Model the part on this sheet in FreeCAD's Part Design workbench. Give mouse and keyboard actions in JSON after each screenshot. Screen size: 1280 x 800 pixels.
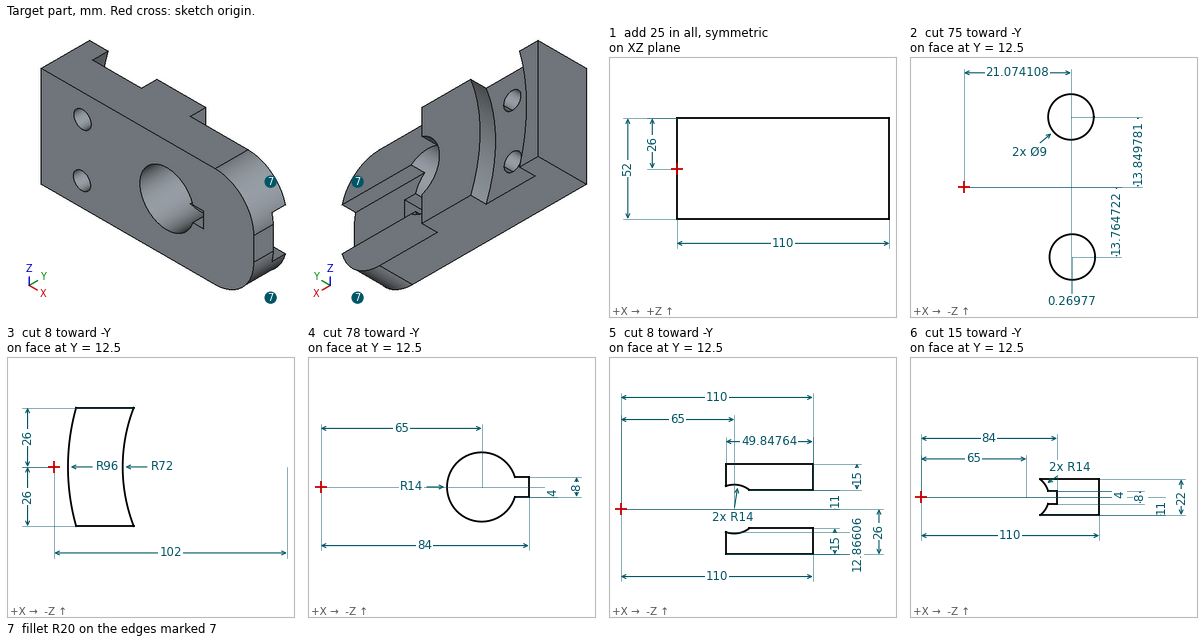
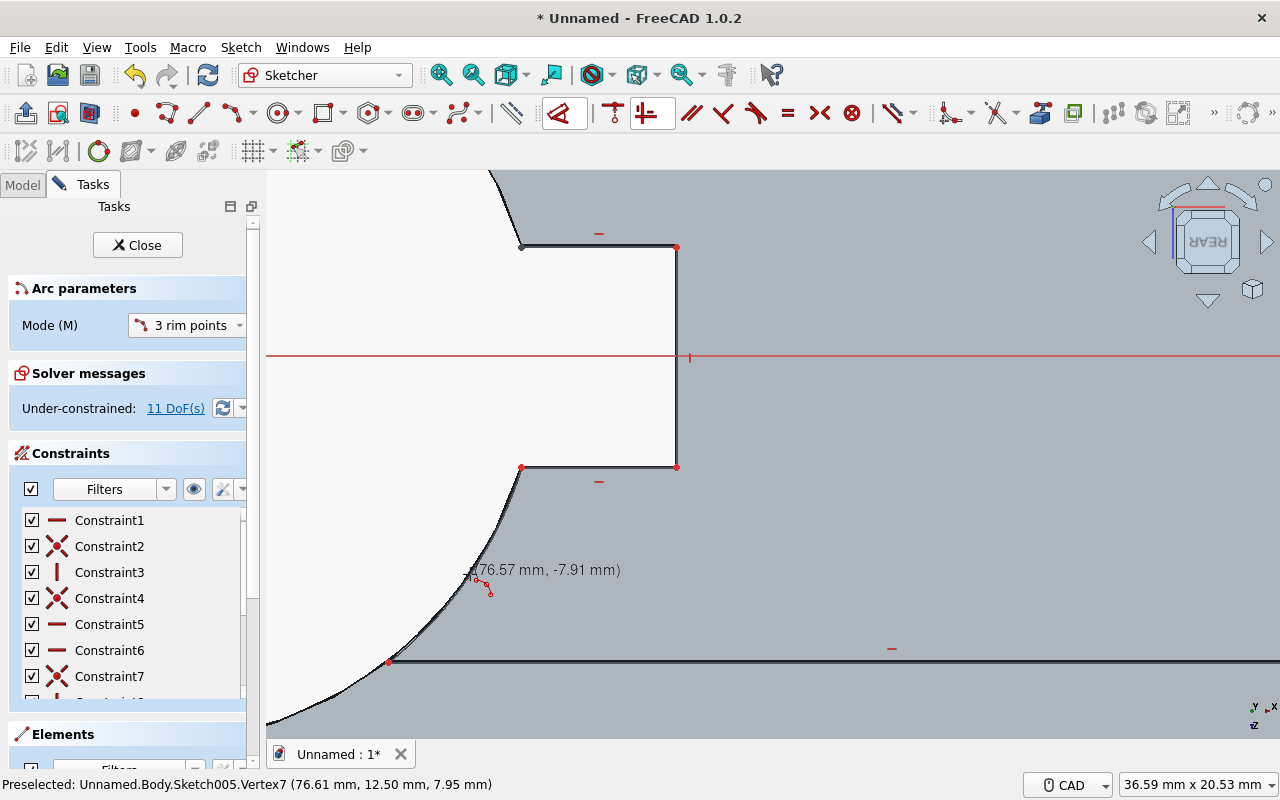
{"action": "scroll", "coordinate": [475, 575], "scroll_direction": "down", "scroll_amount": 3}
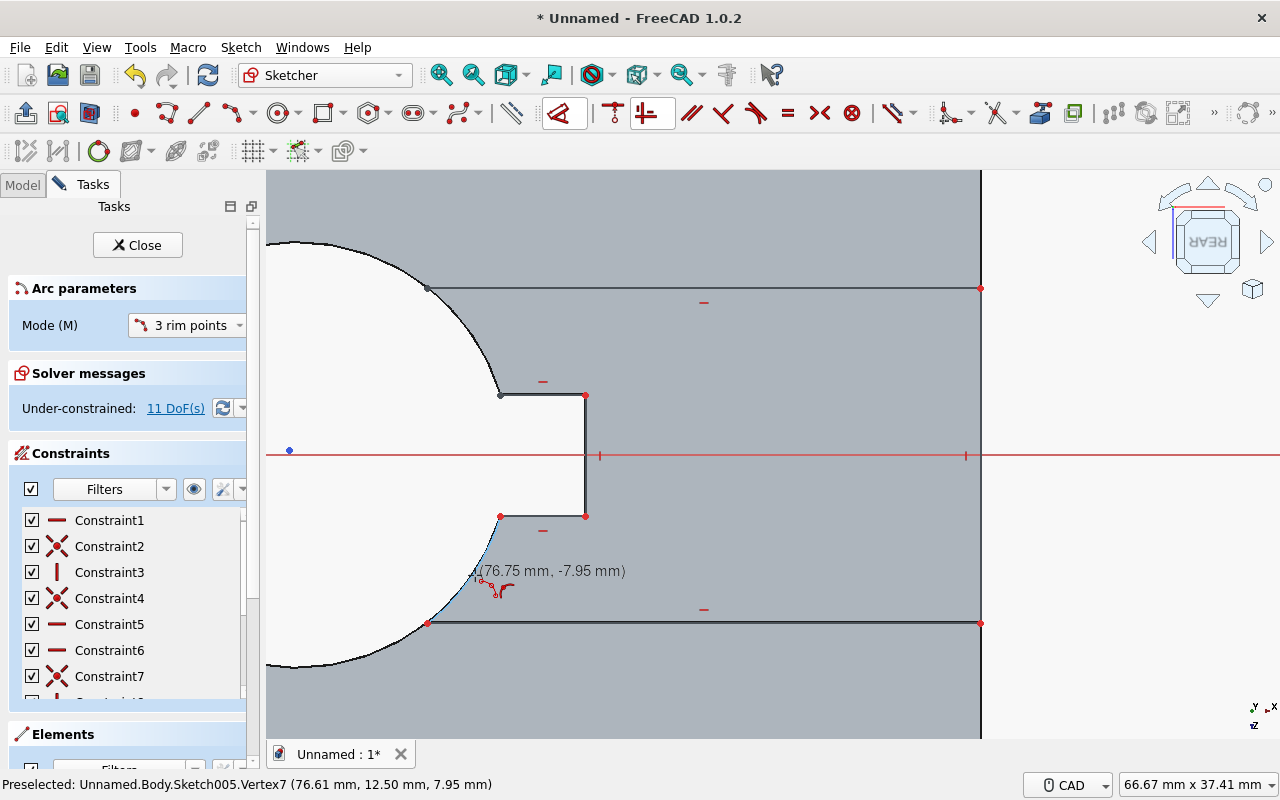
{"action": "left_click", "coordinate": [428, 288]}
{"action": "left_click", "coordinate": [501, 395]}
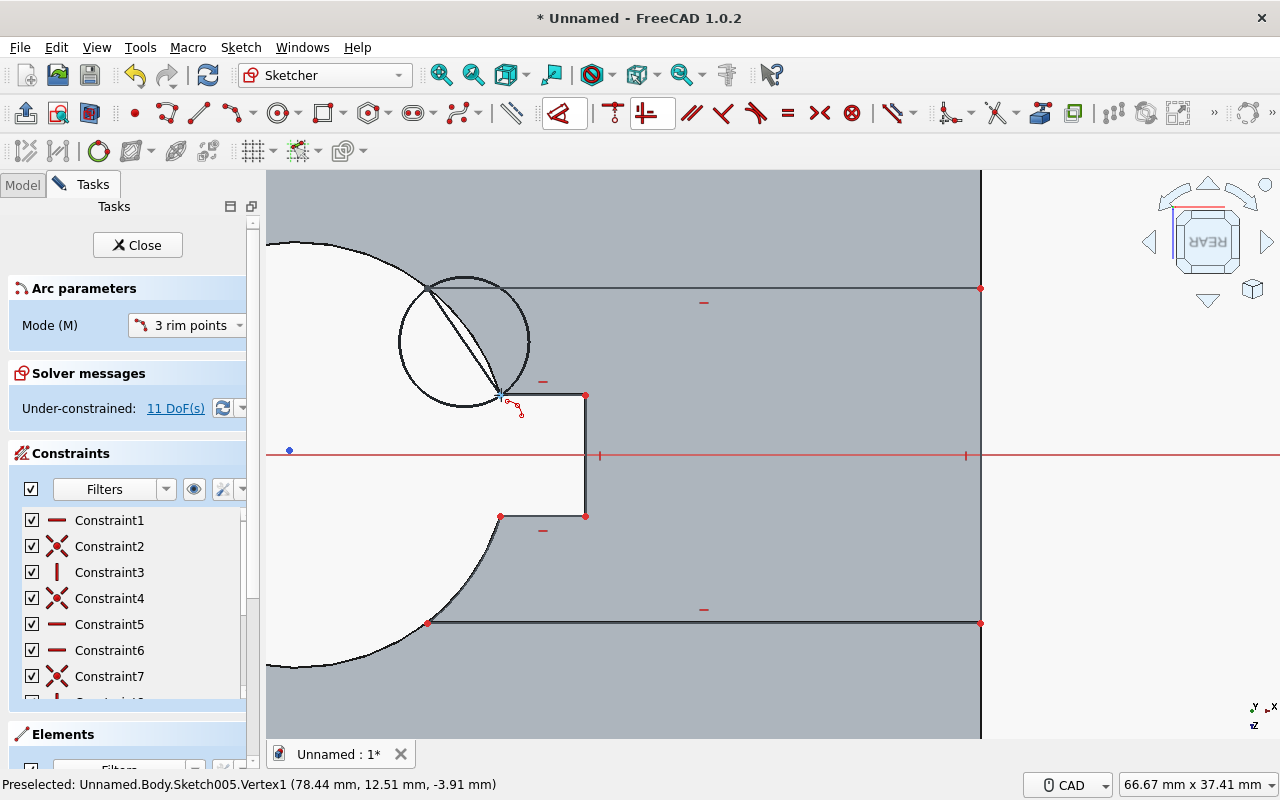
{"action": "scroll", "coordinate": [472, 335], "scroll_direction": "up", "scroll_amount": 3}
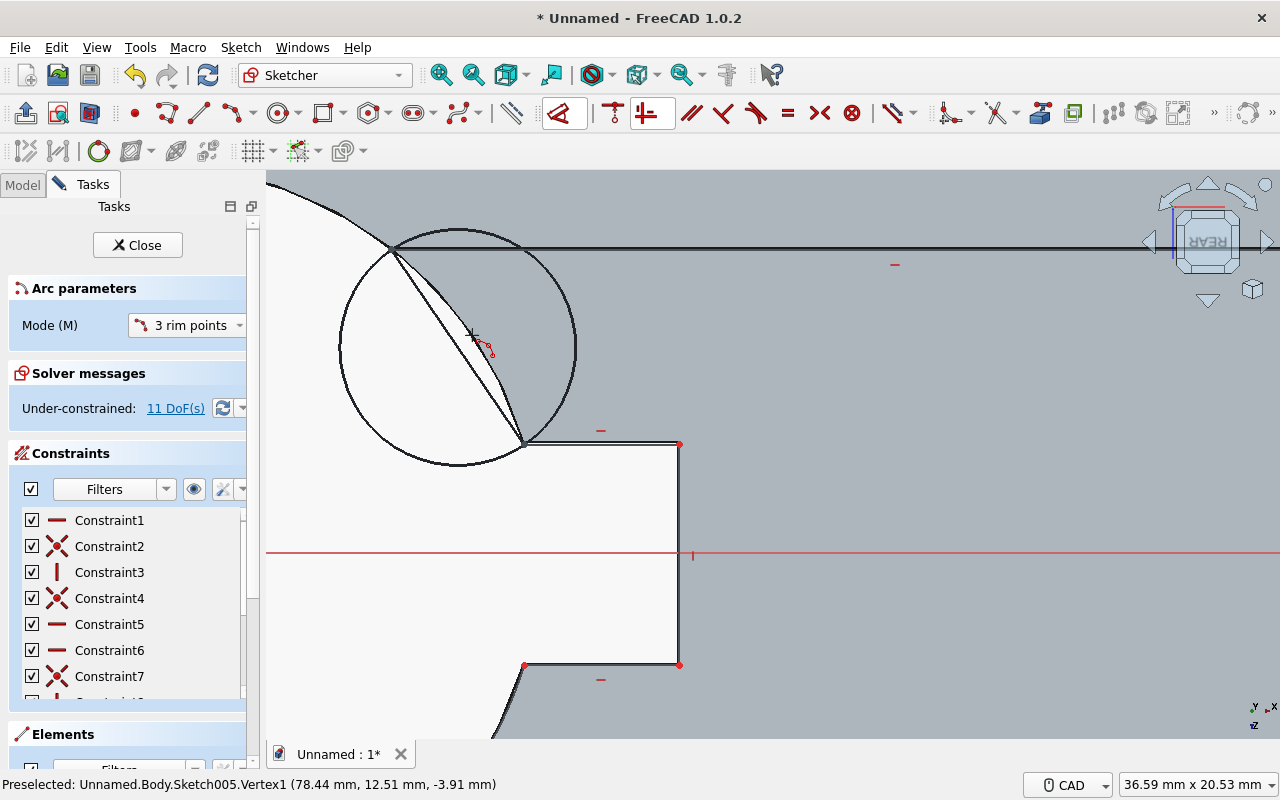
{"action": "left_click", "coordinate": [473, 335]}
{"action": "key", "text": "Escape"}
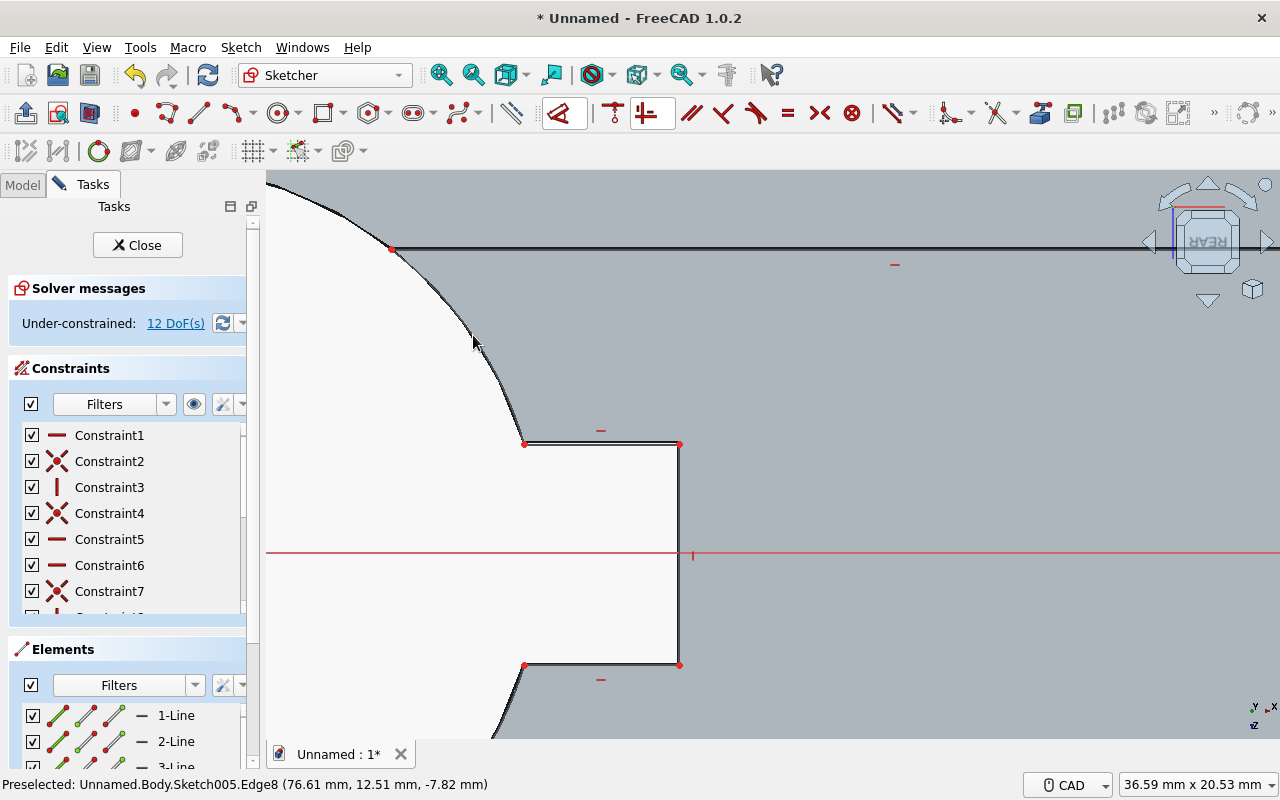
{"action": "left_click", "coordinate": [507, 710]}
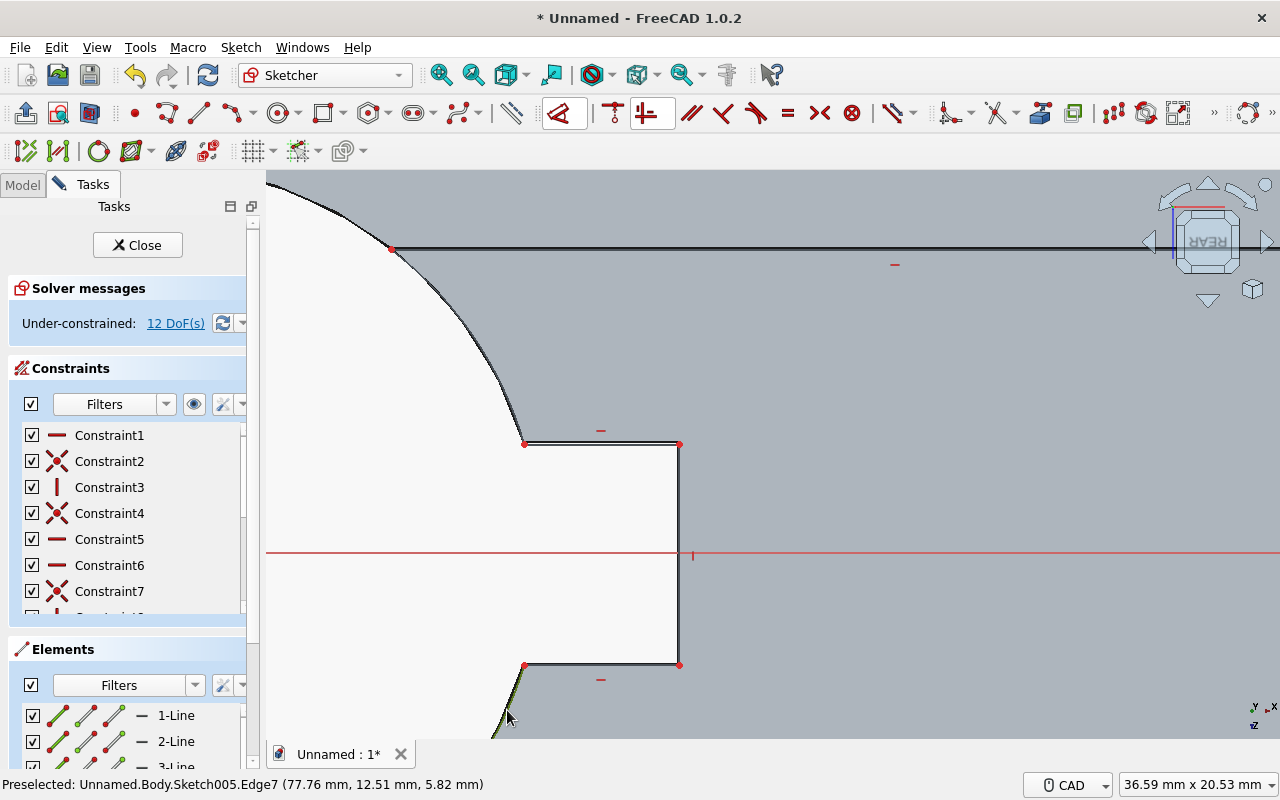
{"action": "left_click", "coordinate": [498, 378]}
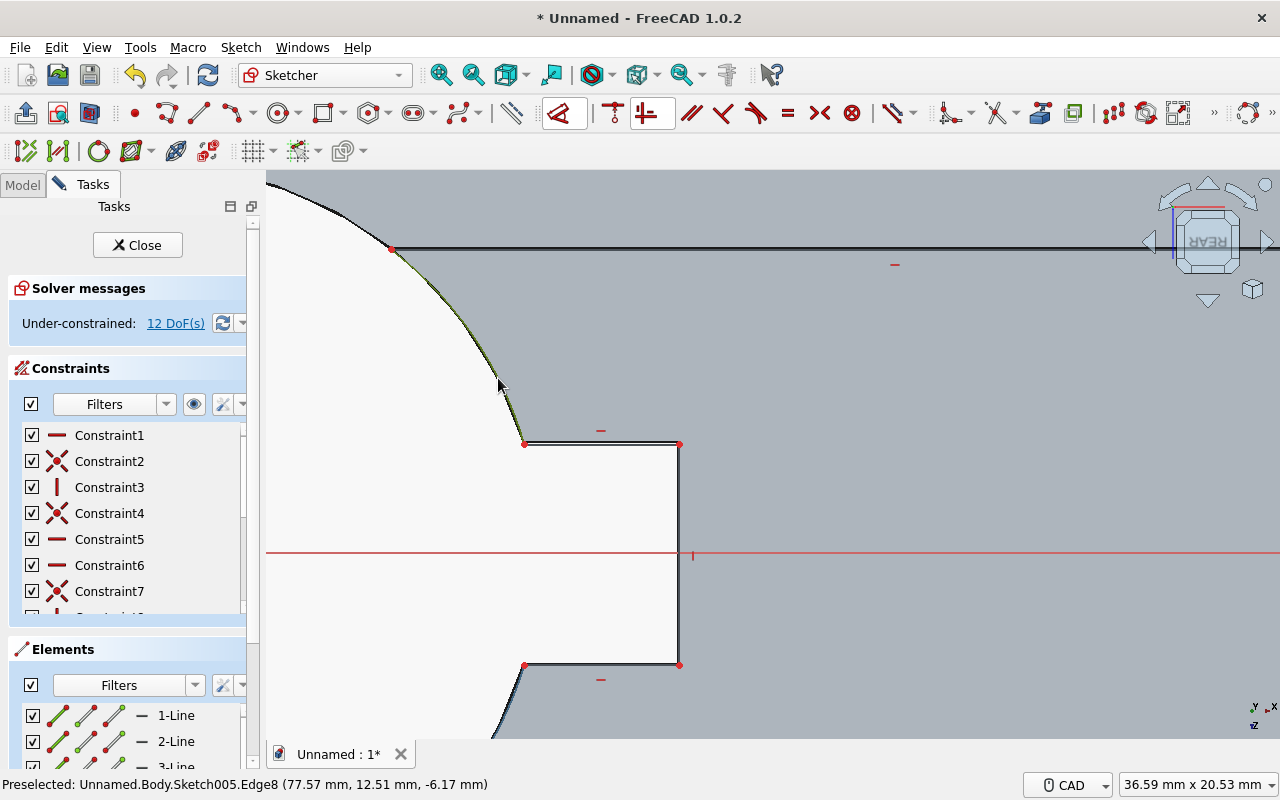
{"action": "left_click", "coordinate": [614, 114]}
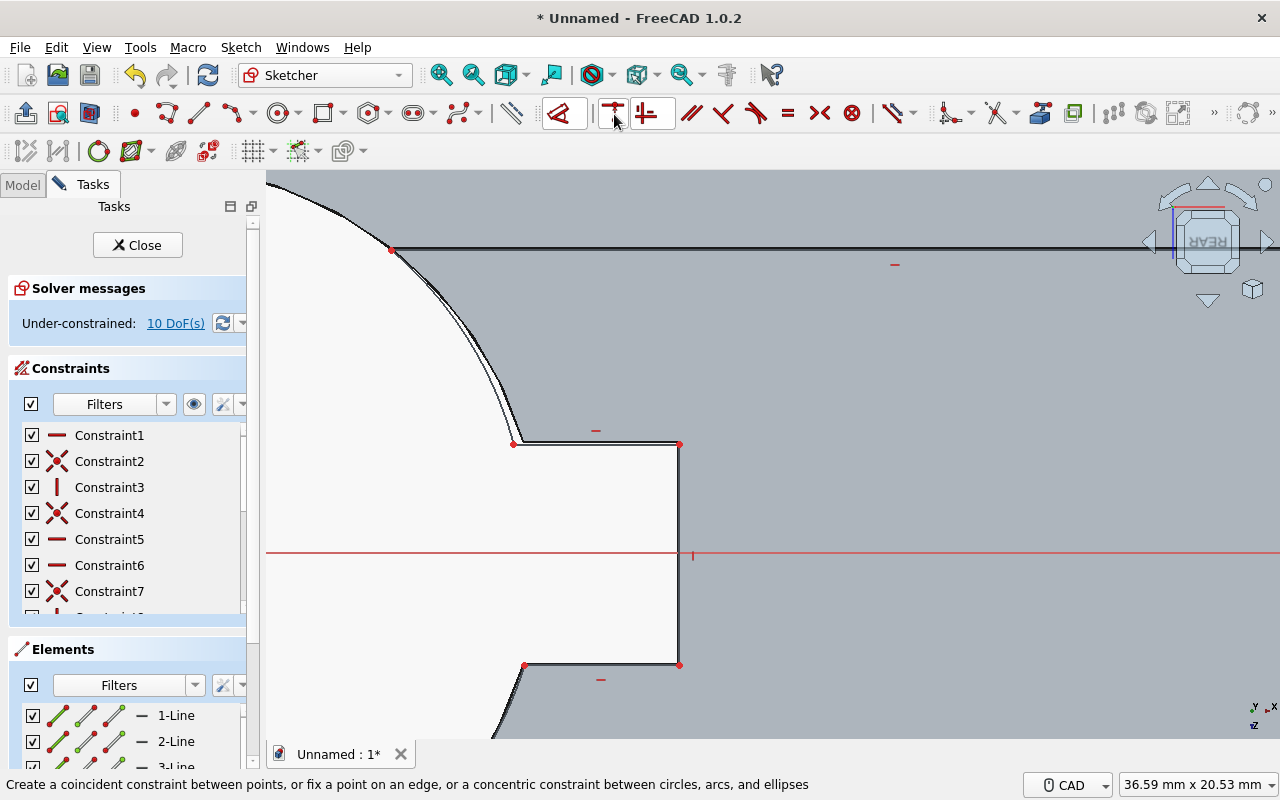
{"action": "left_click", "coordinate": [508, 710]}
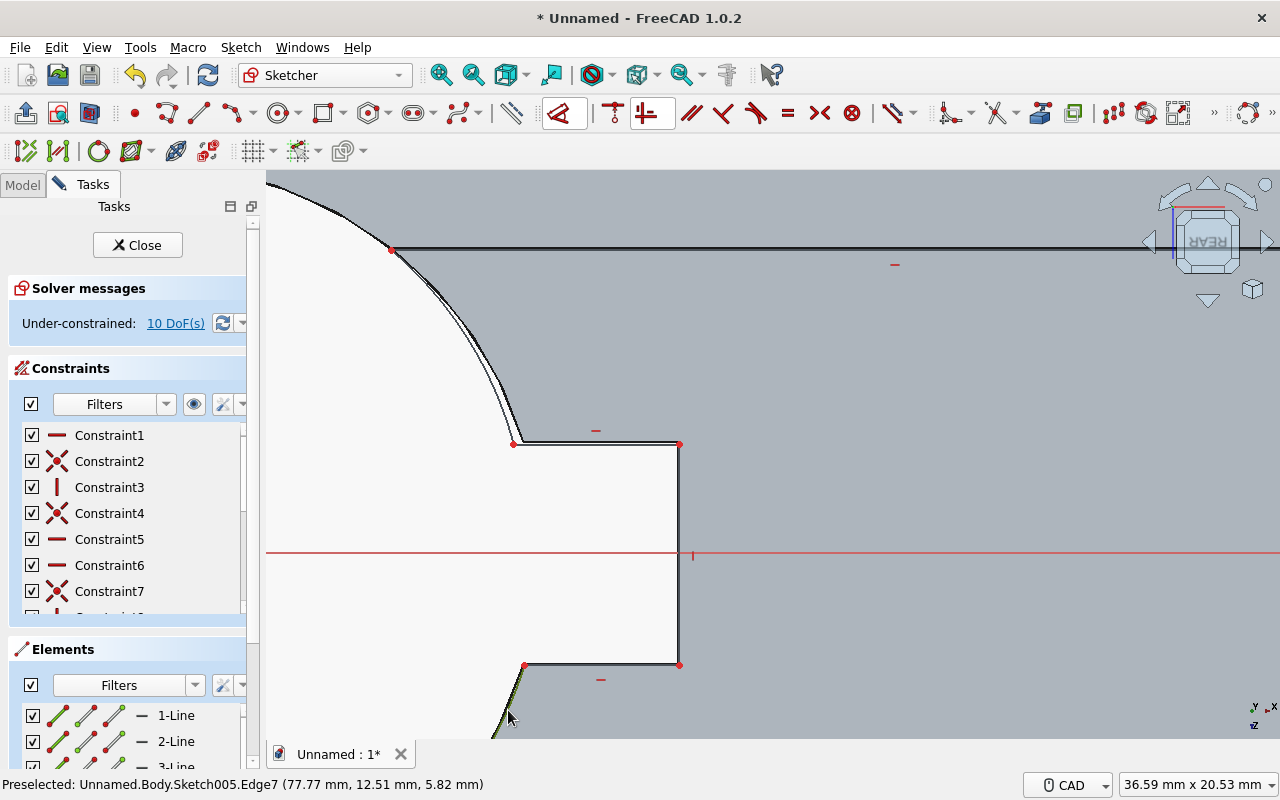
{"action": "left_click", "coordinate": [490, 379]}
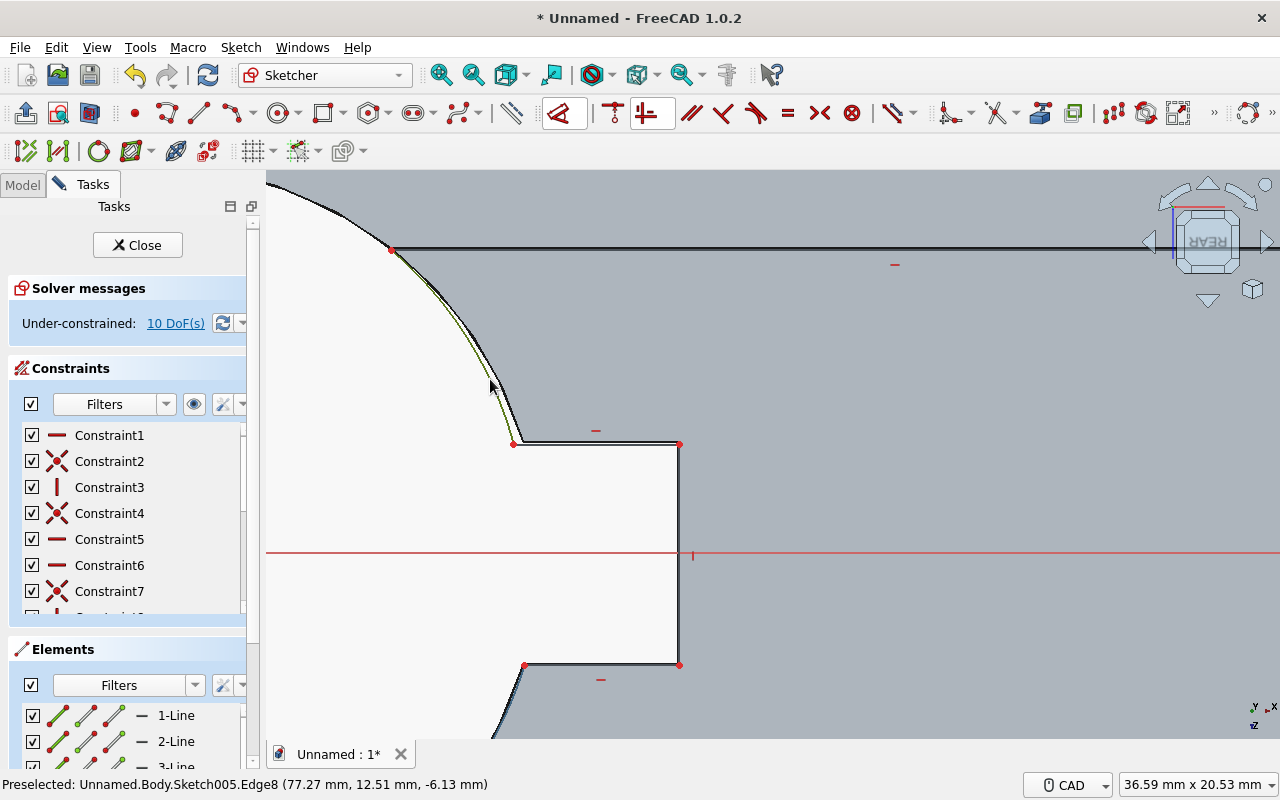
{"action": "left_click", "coordinate": [788, 114]}